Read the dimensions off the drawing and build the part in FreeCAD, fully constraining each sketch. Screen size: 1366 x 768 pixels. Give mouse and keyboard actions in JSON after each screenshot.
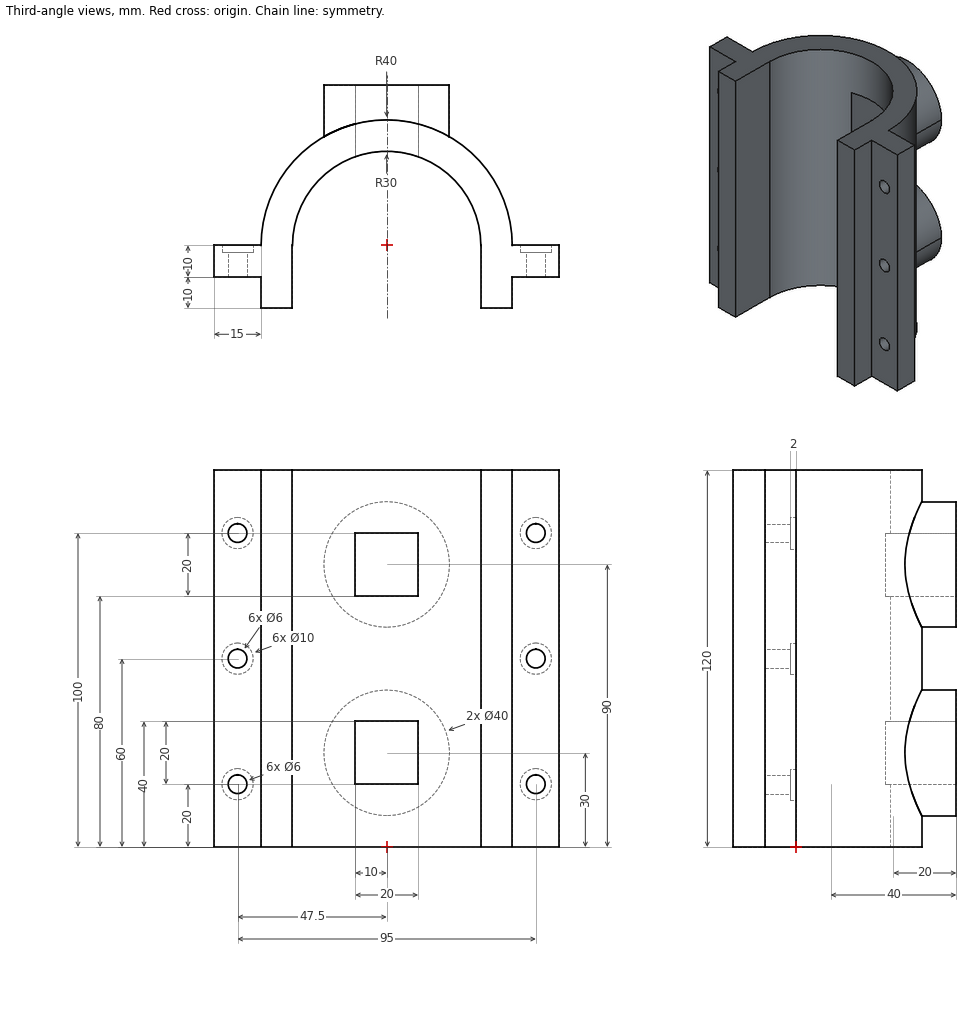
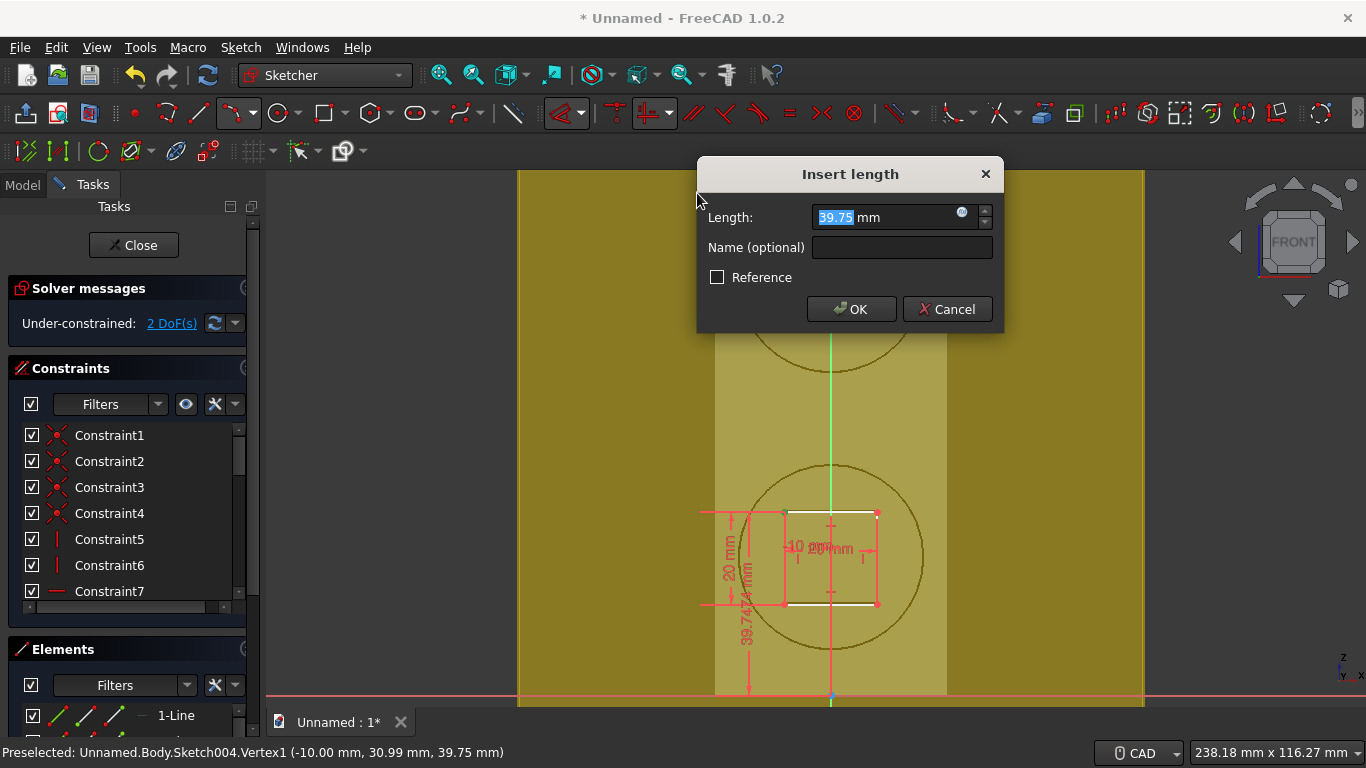
{"action": "type", "text": "40"}
{"action": "key", "text": "Return"}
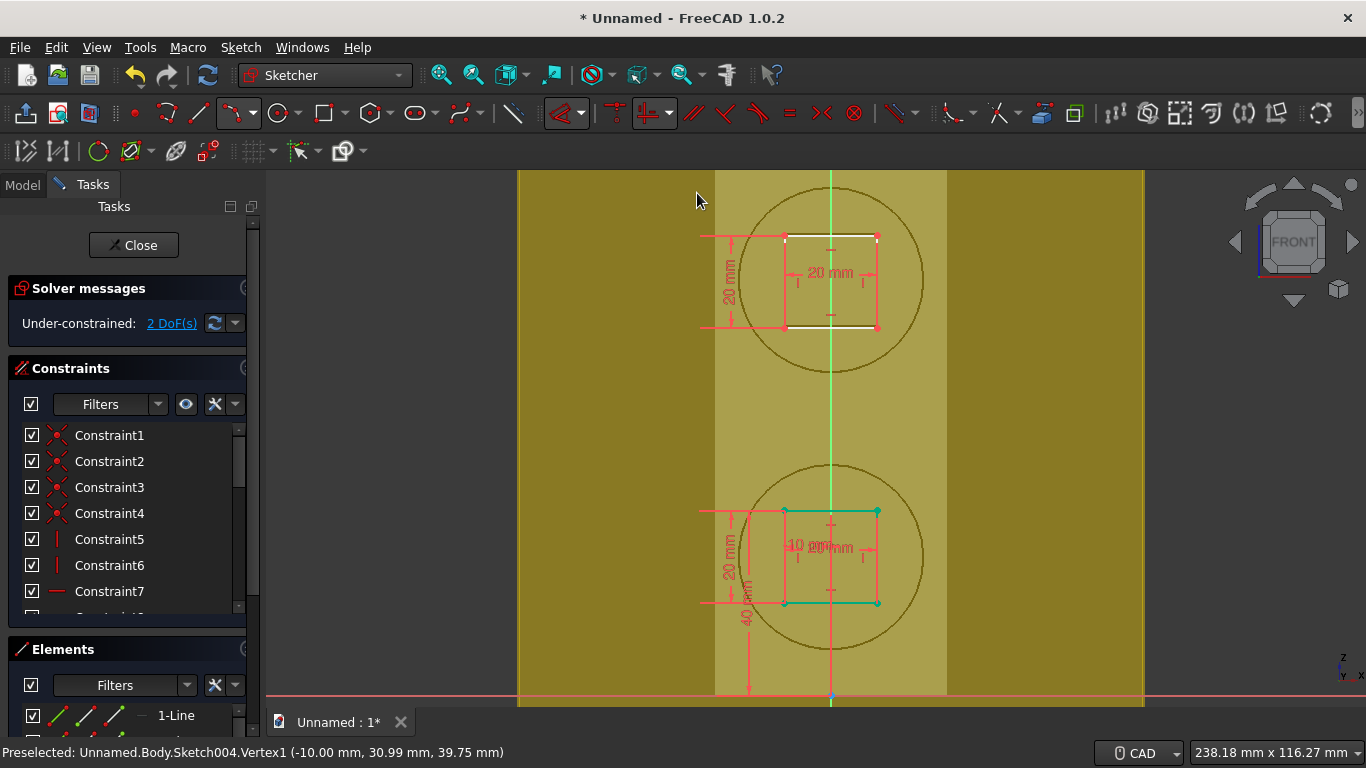
{"action": "left_click", "coordinate": [785, 236]}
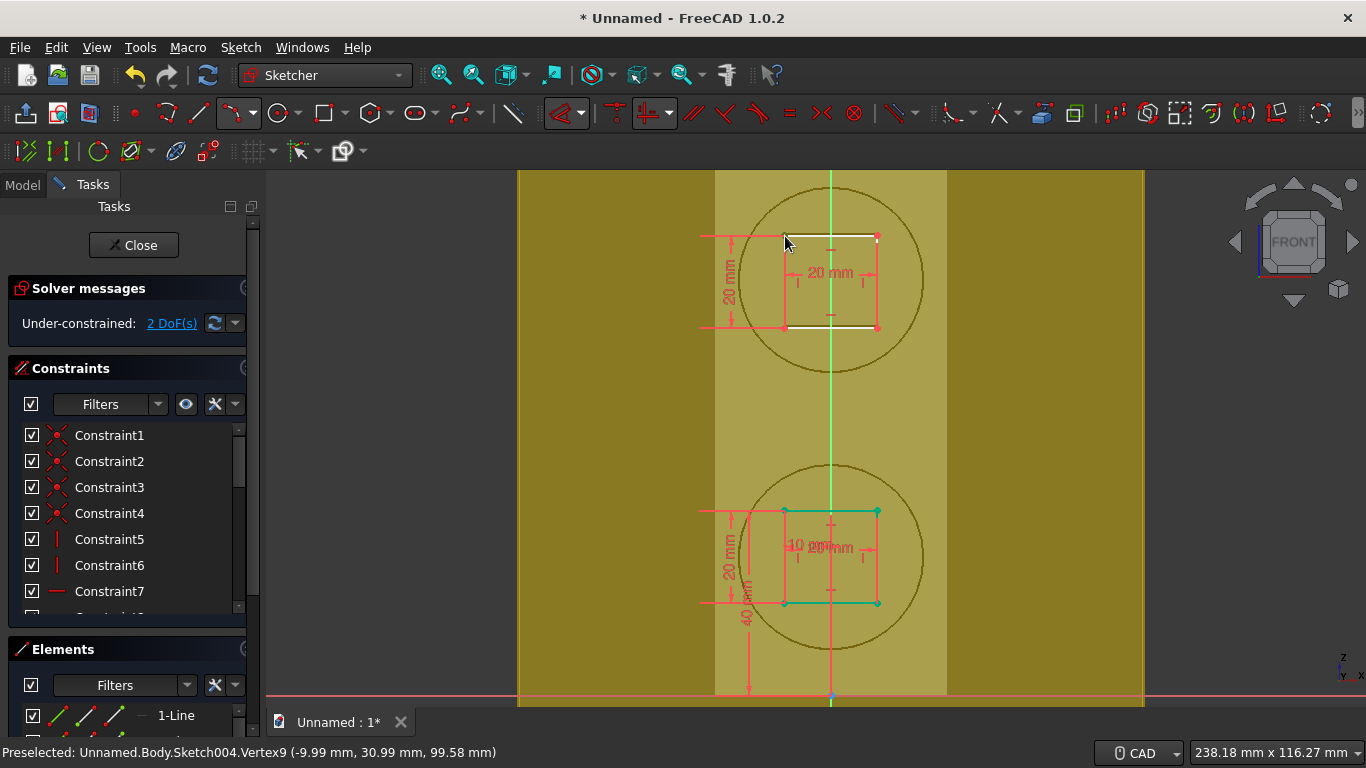
{"action": "key", "text": "l"}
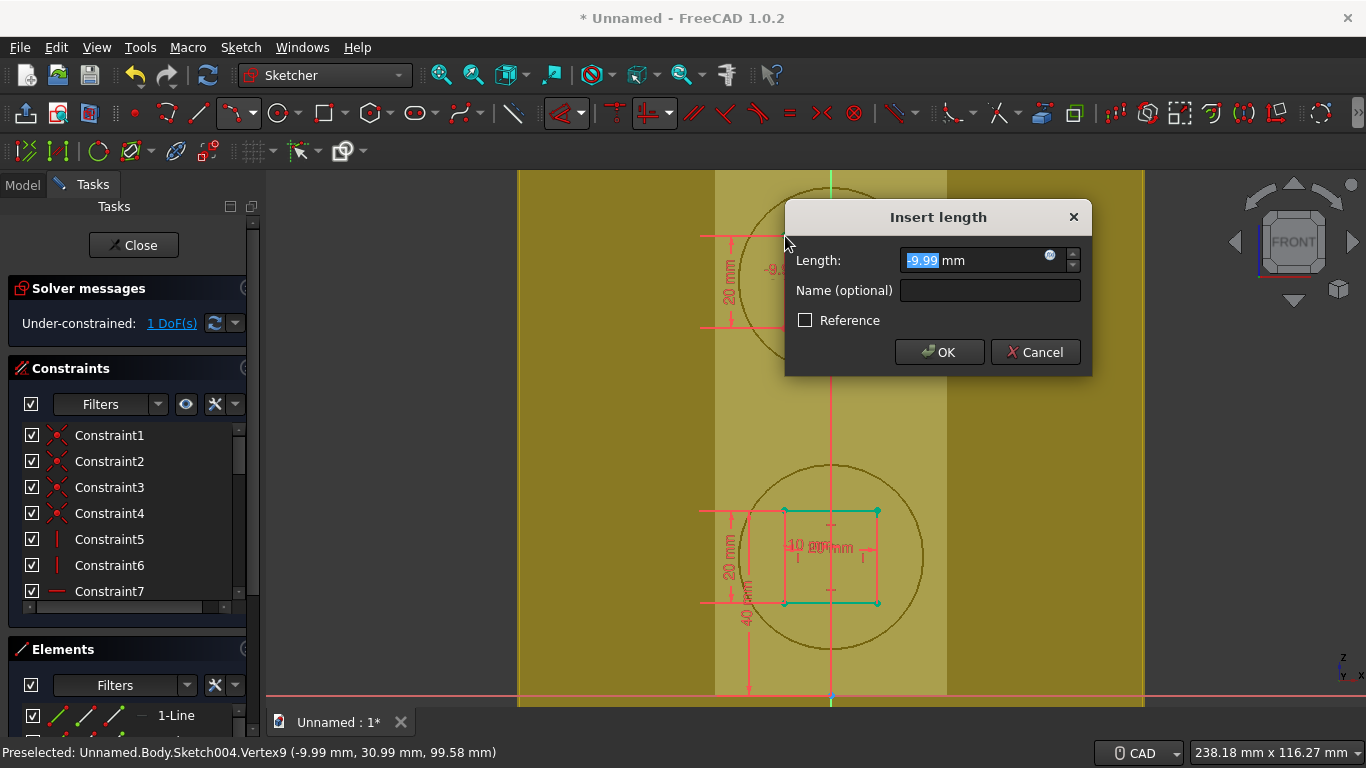
{"action": "type", "text": "-10"}
{"action": "key", "text": "Return"}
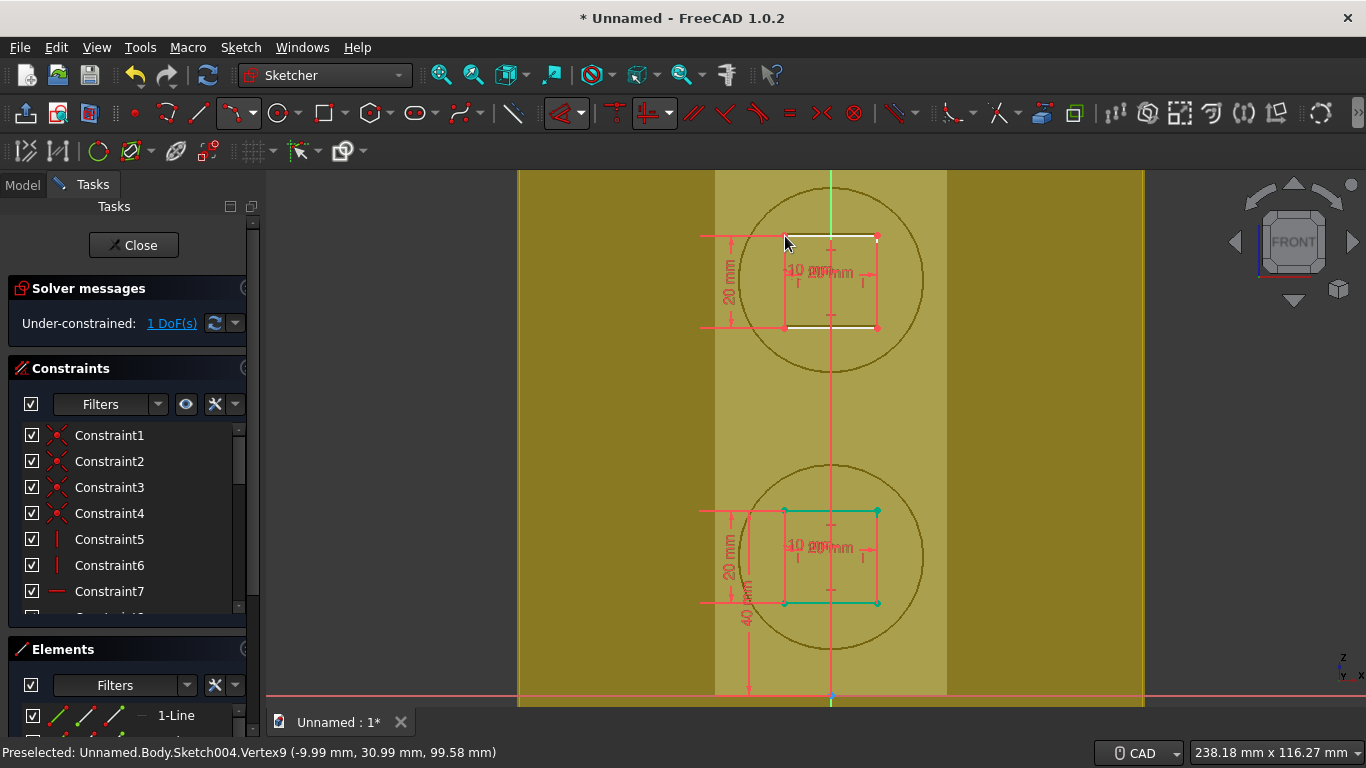
{"action": "left_click", "coordinate": [785, 328]}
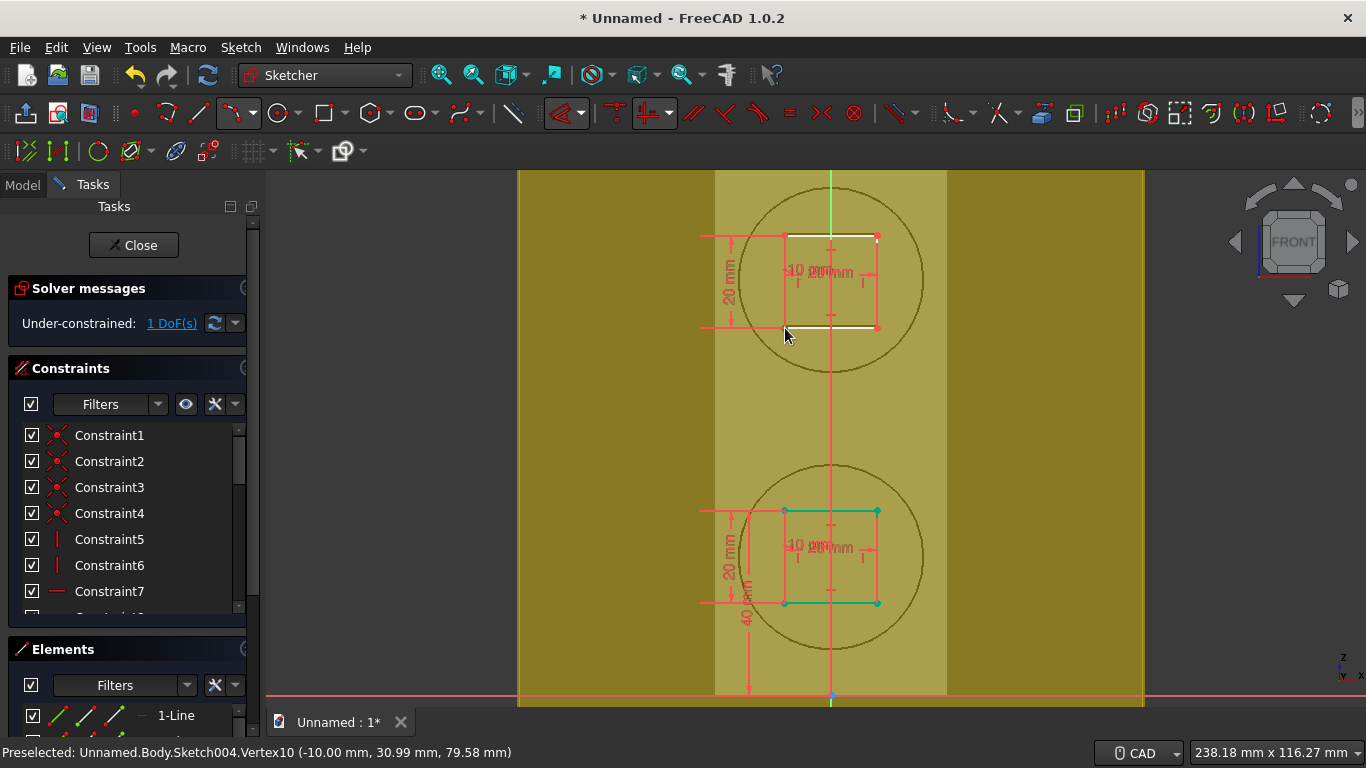
{"action": "key", "text": "i"}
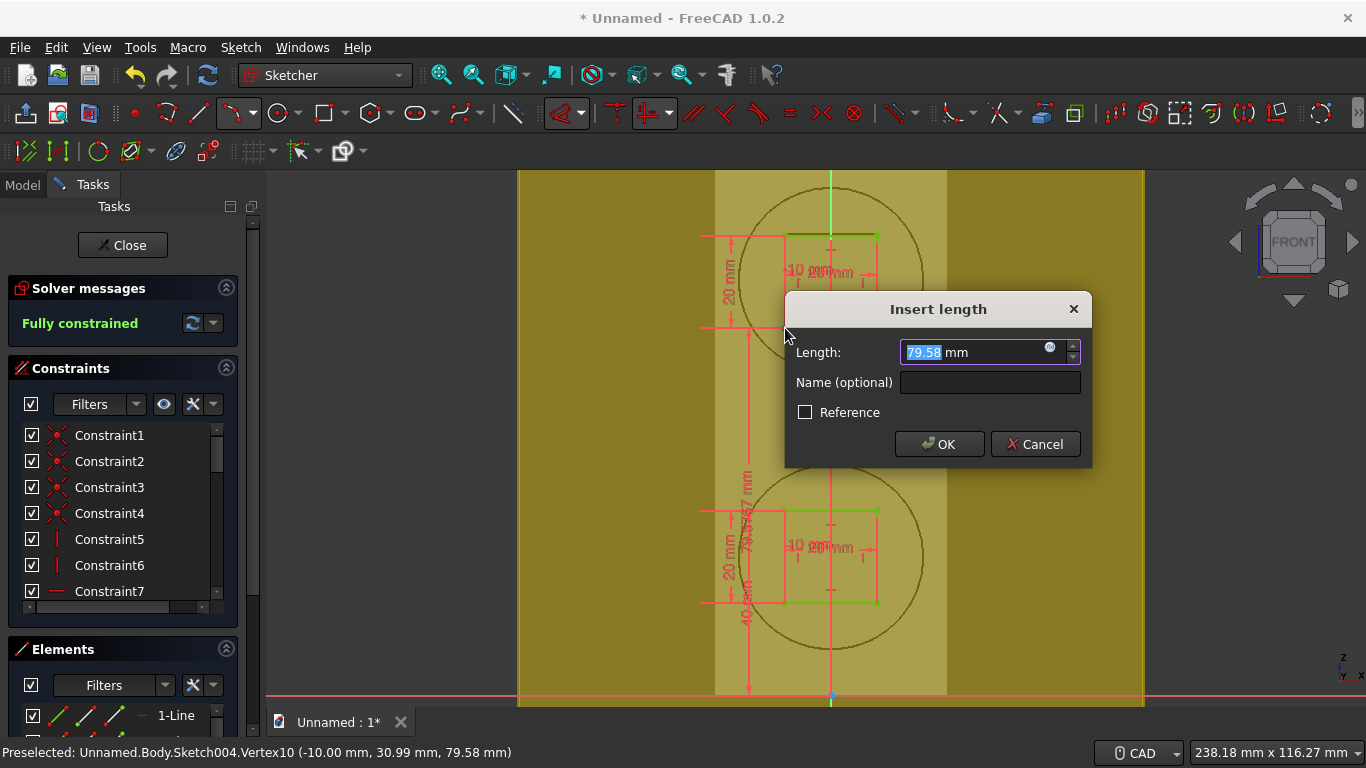
{"action": "type", "text": "80"}
{"action": "key", "text": "Return"}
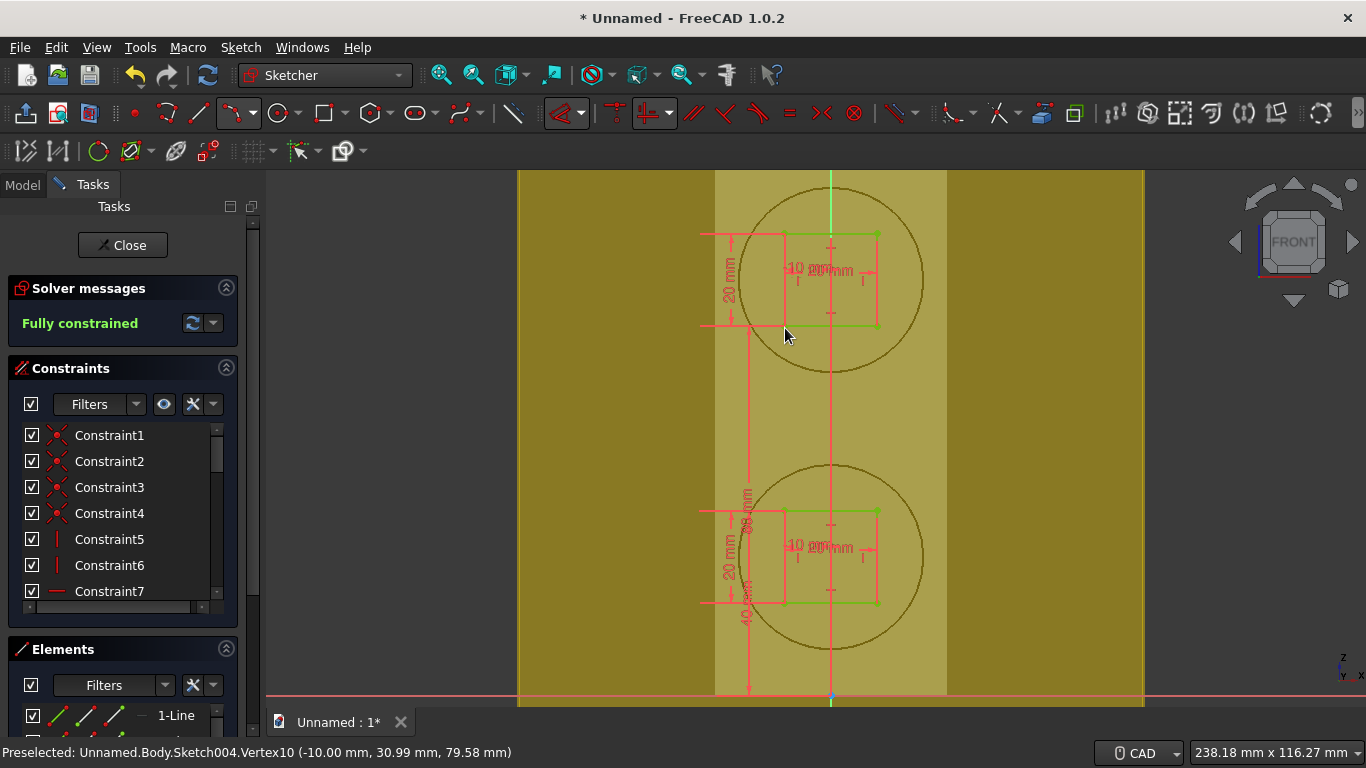
{"action": "left_click", "coordinate": [123, 245]}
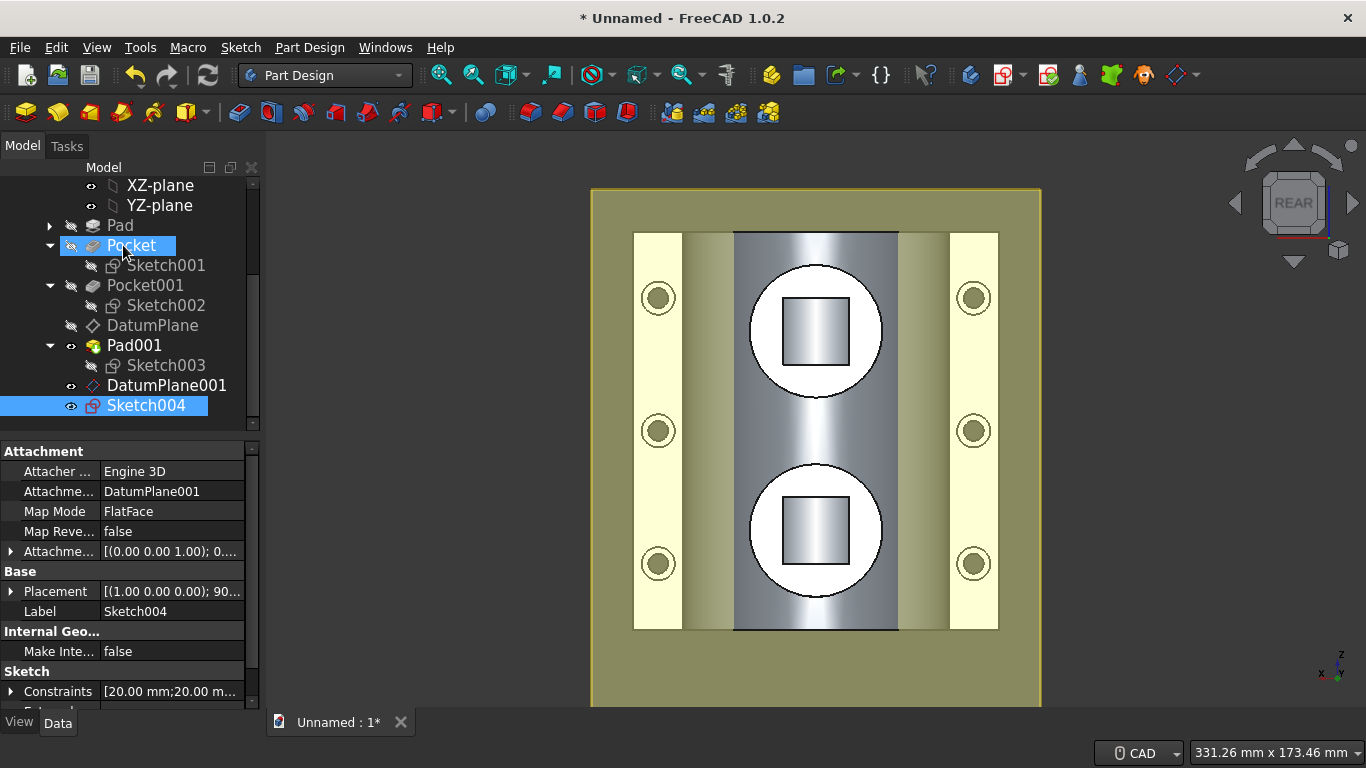
{"action": "left_click", "coordinate": [240, 112]}